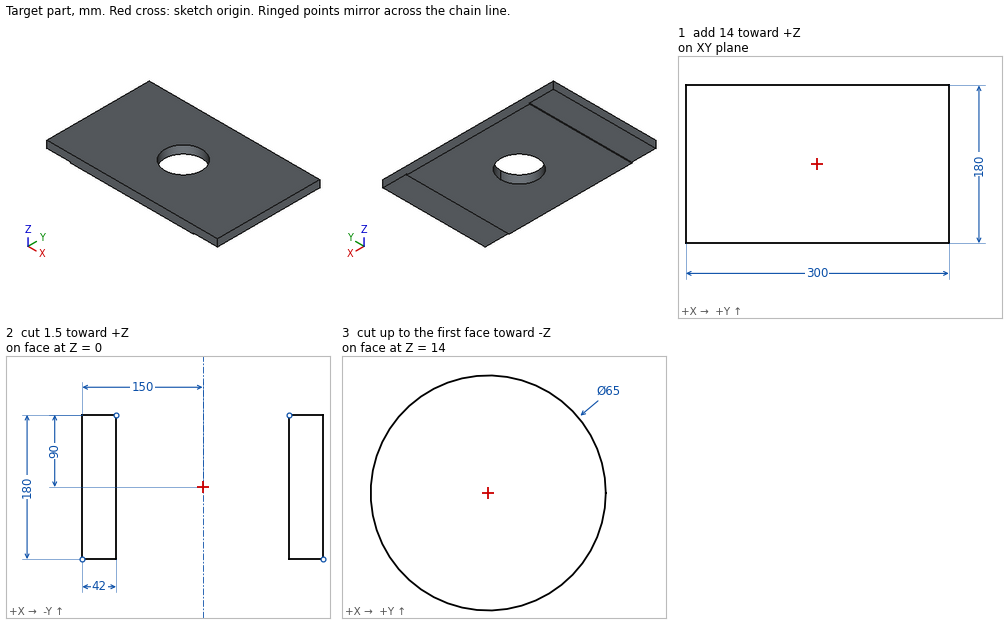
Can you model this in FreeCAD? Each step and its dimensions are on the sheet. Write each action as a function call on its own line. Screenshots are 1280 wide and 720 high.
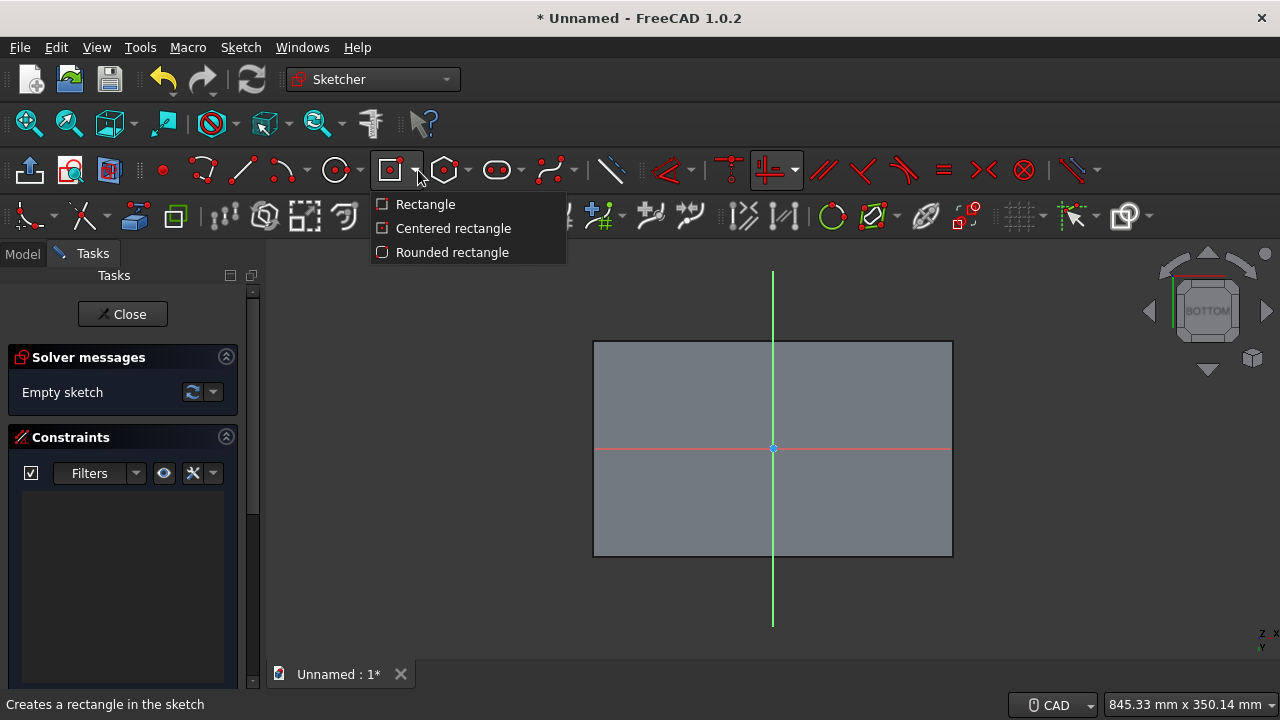
click(468, 204)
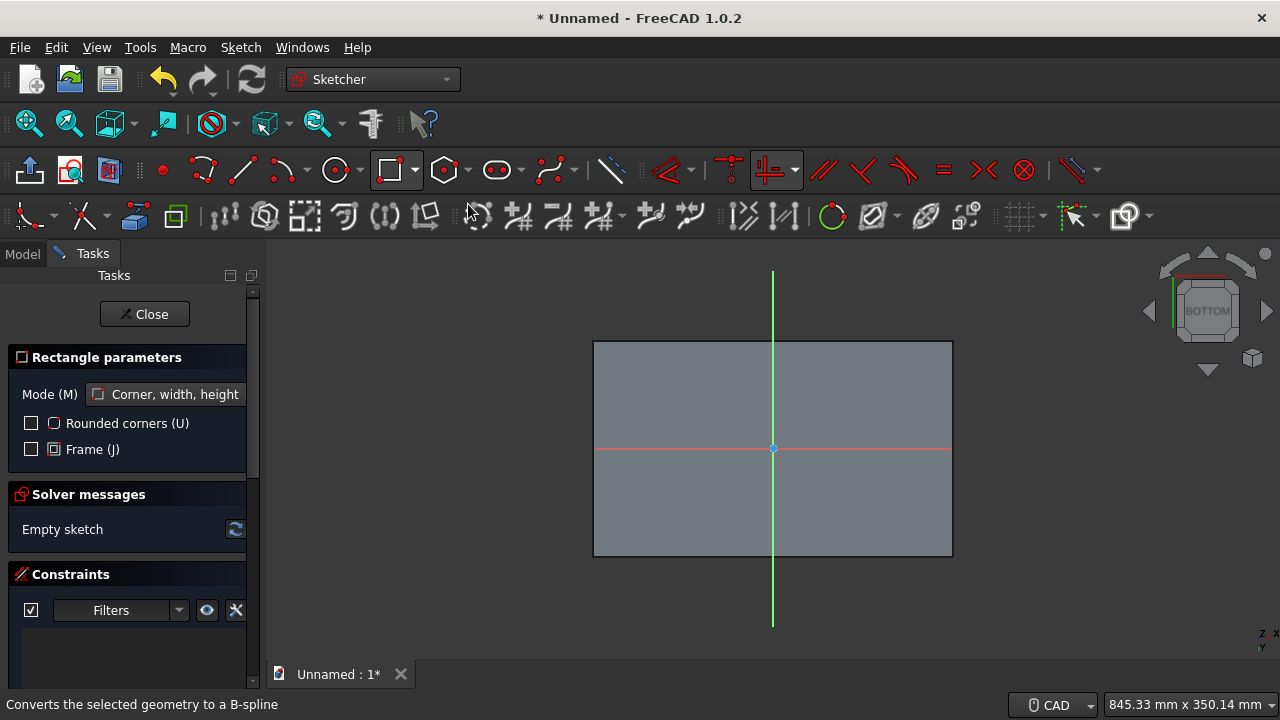
click(593, 341)
click(643, 557)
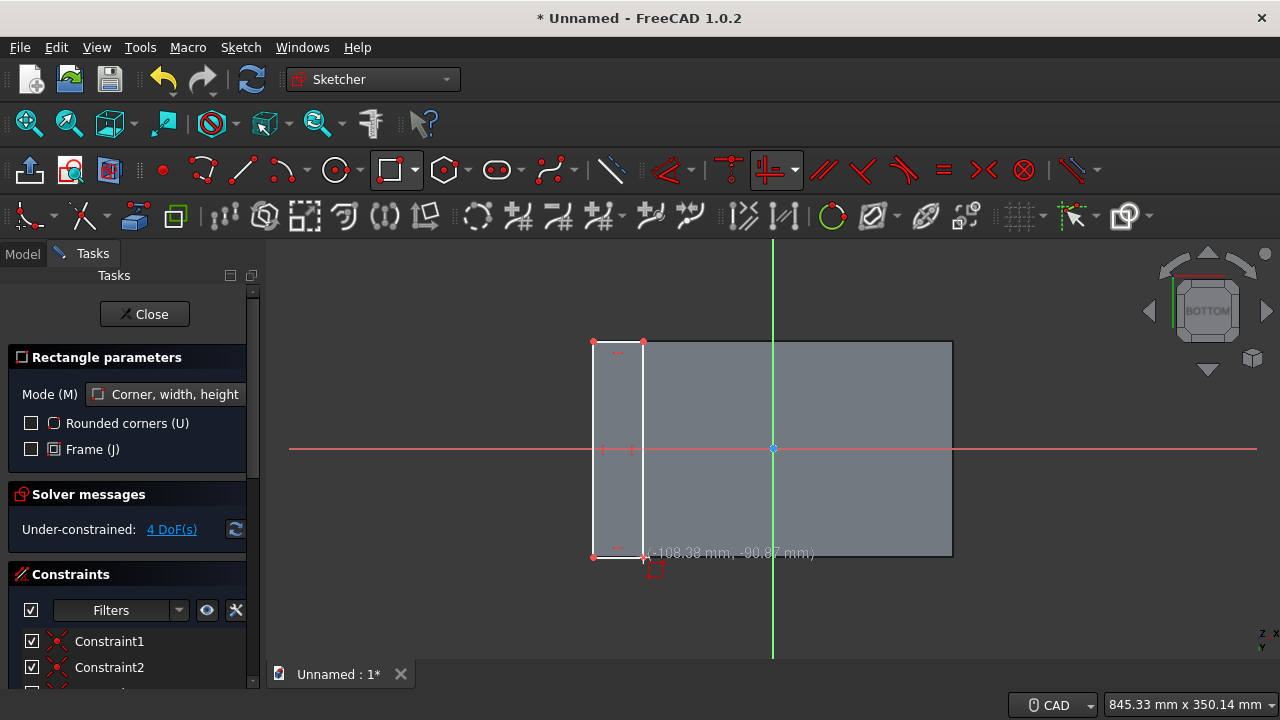
click(903, 341)
click(953, 557)
key(Escape)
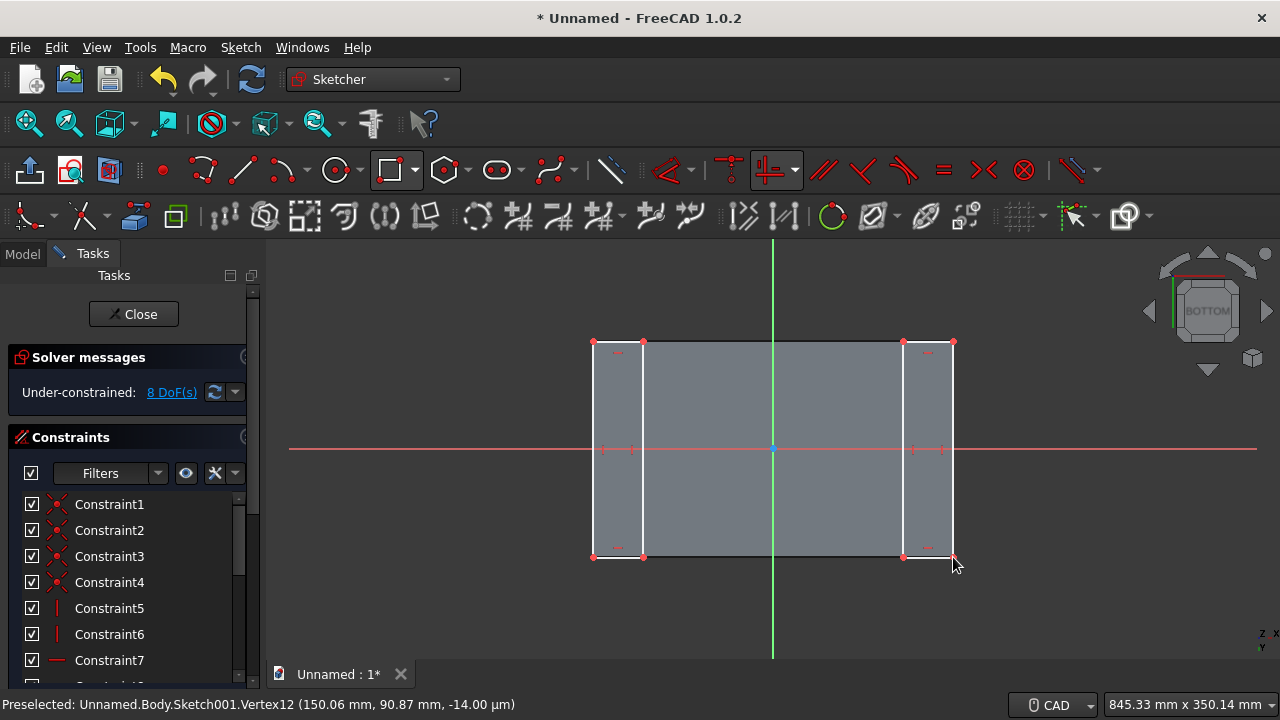
click(643, 342)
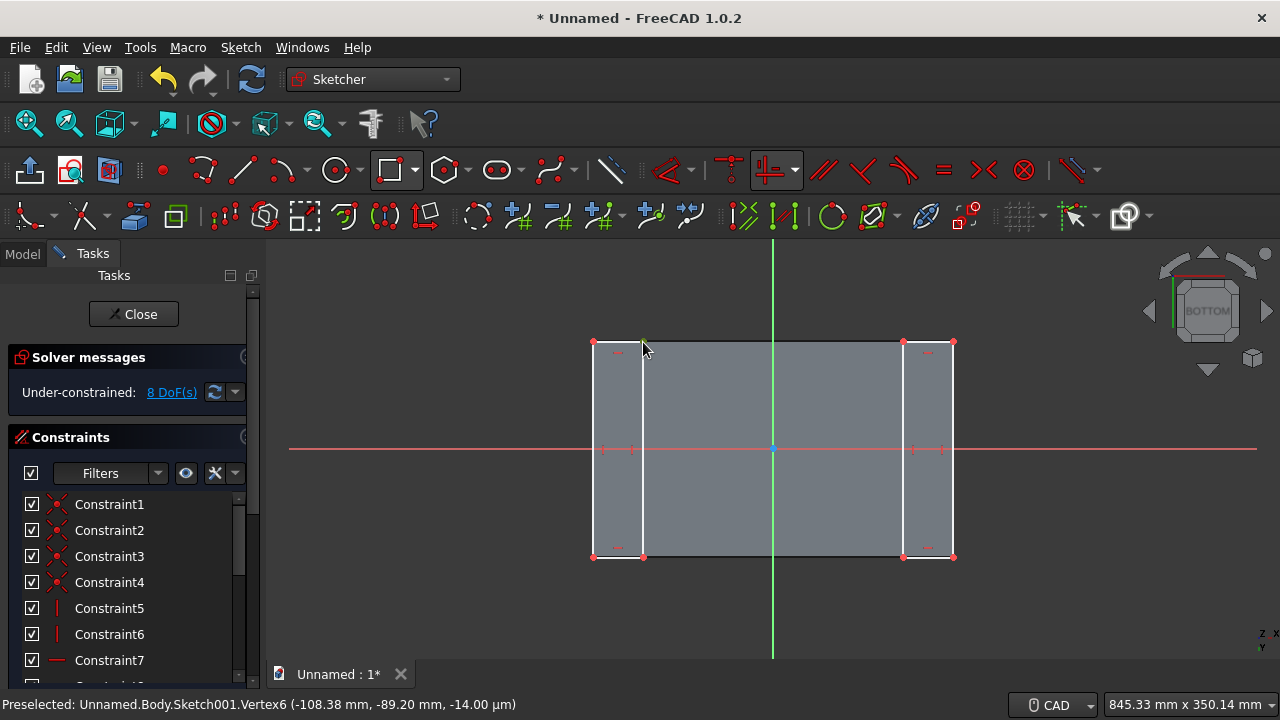
click(903, 342)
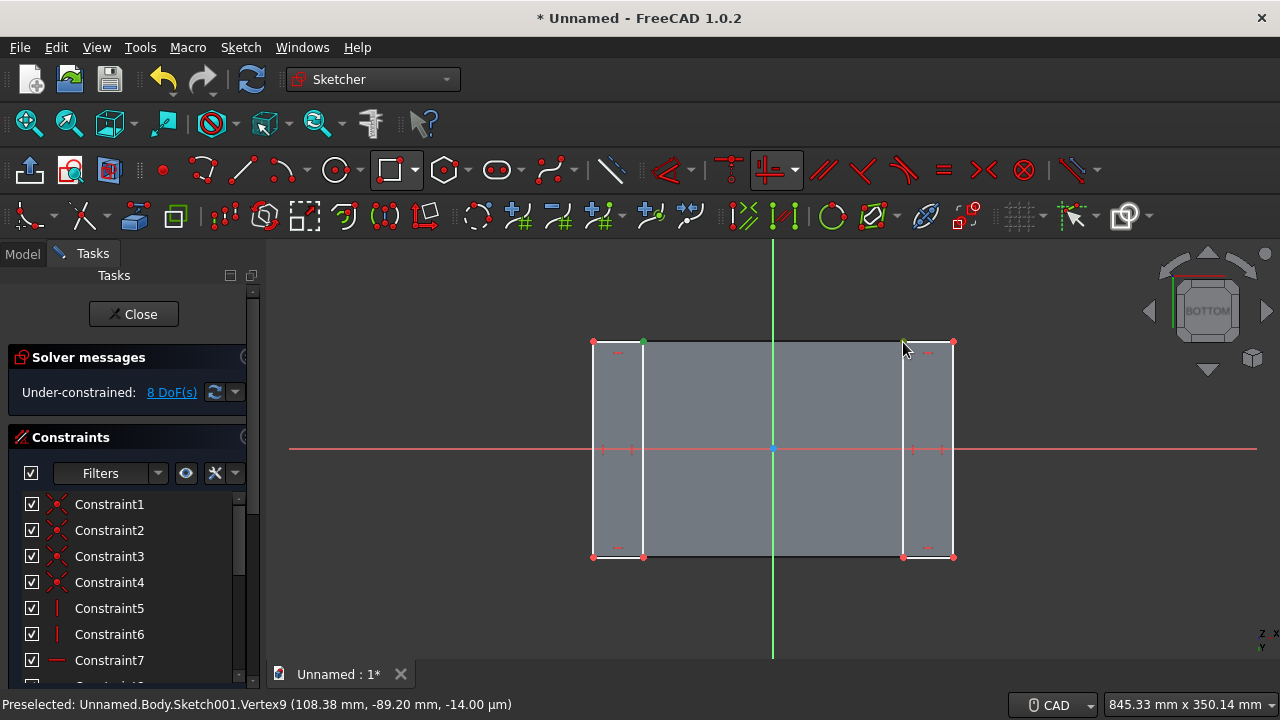
click(773, 605)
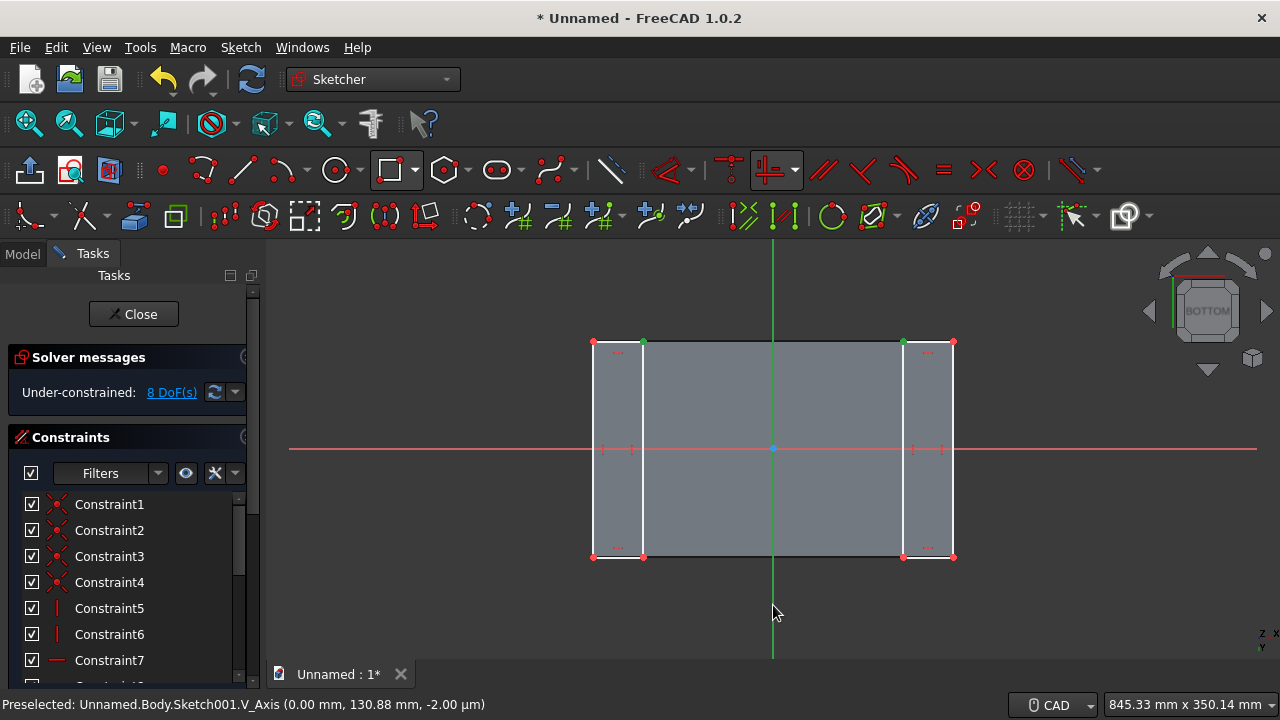
click(984, 170)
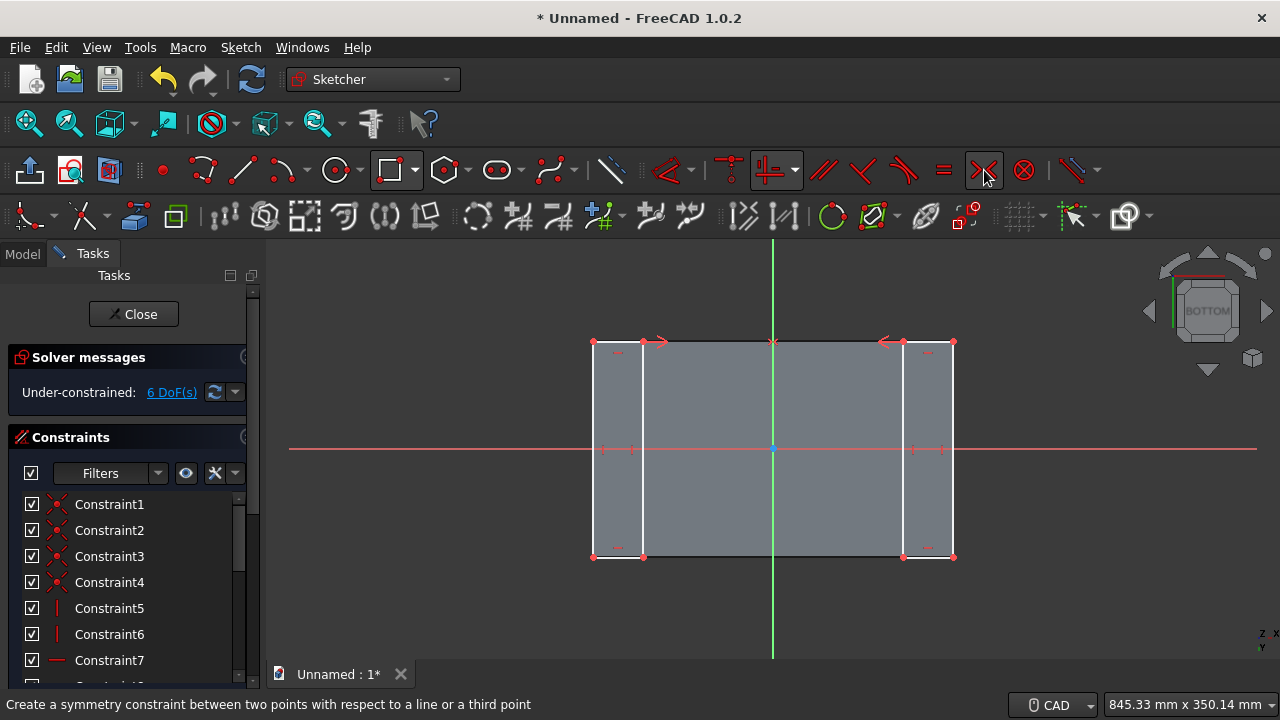
click(593, 558)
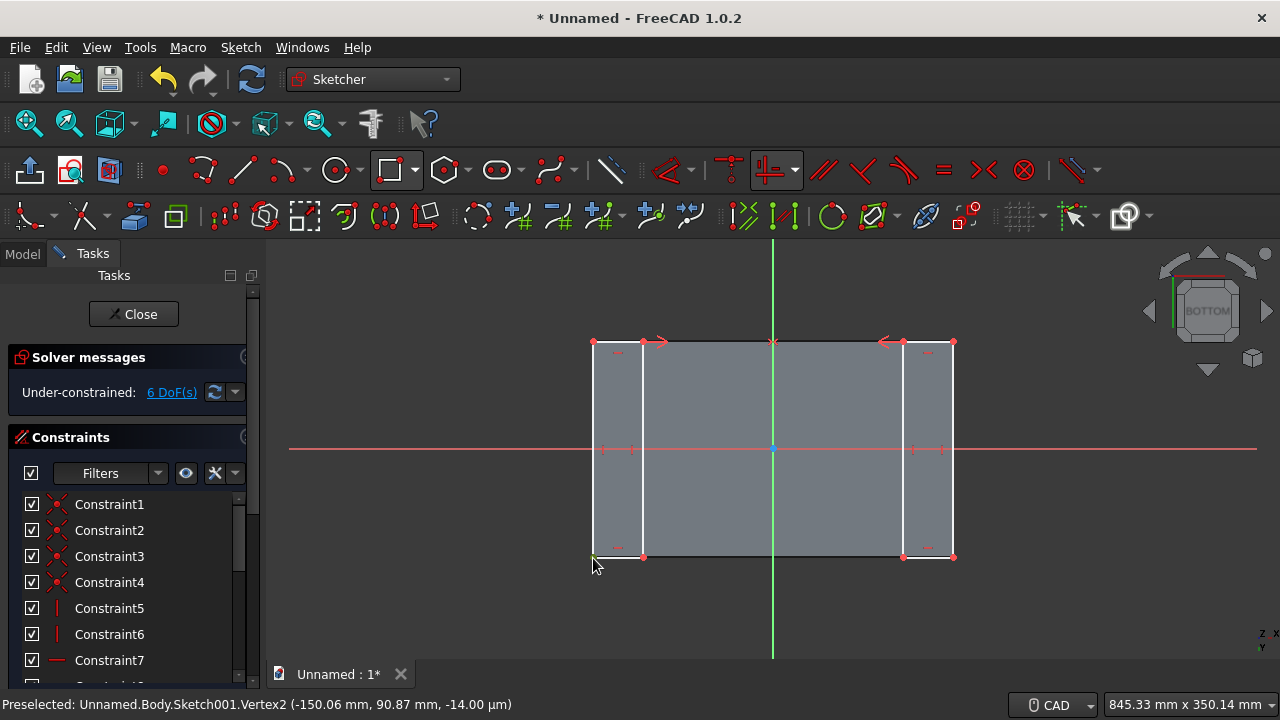
click(953, 558)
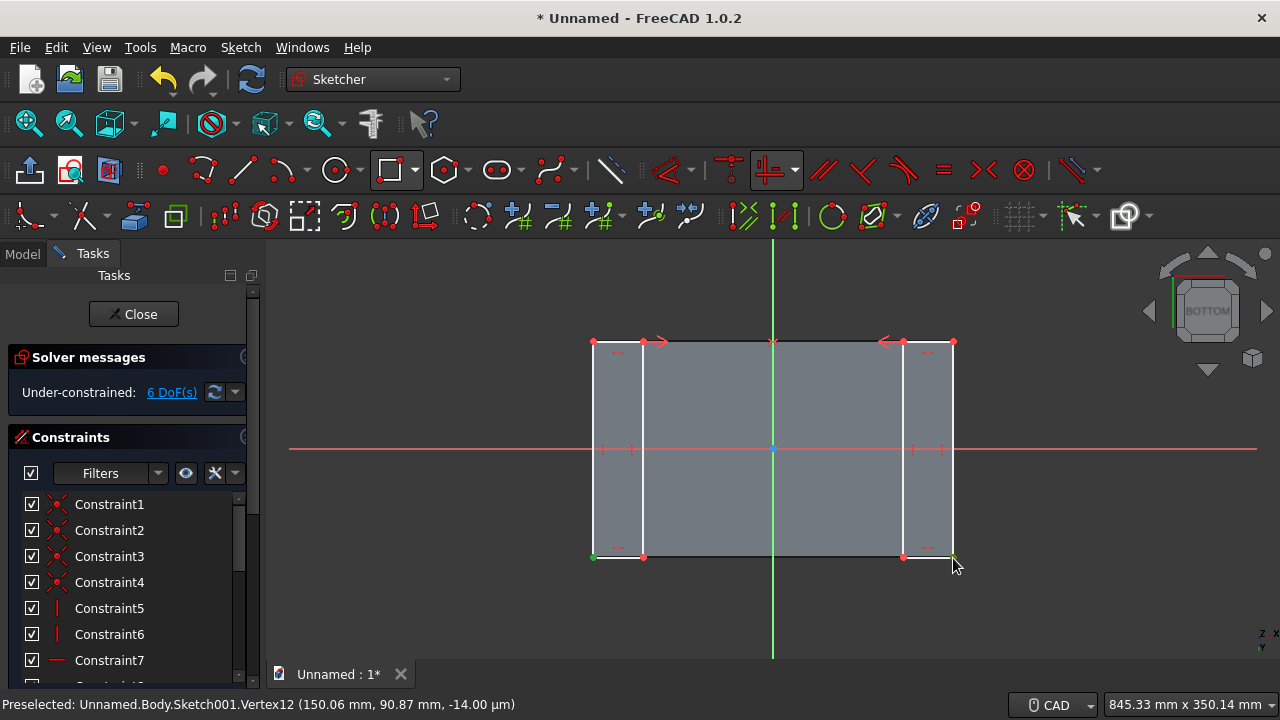
click(773, 605)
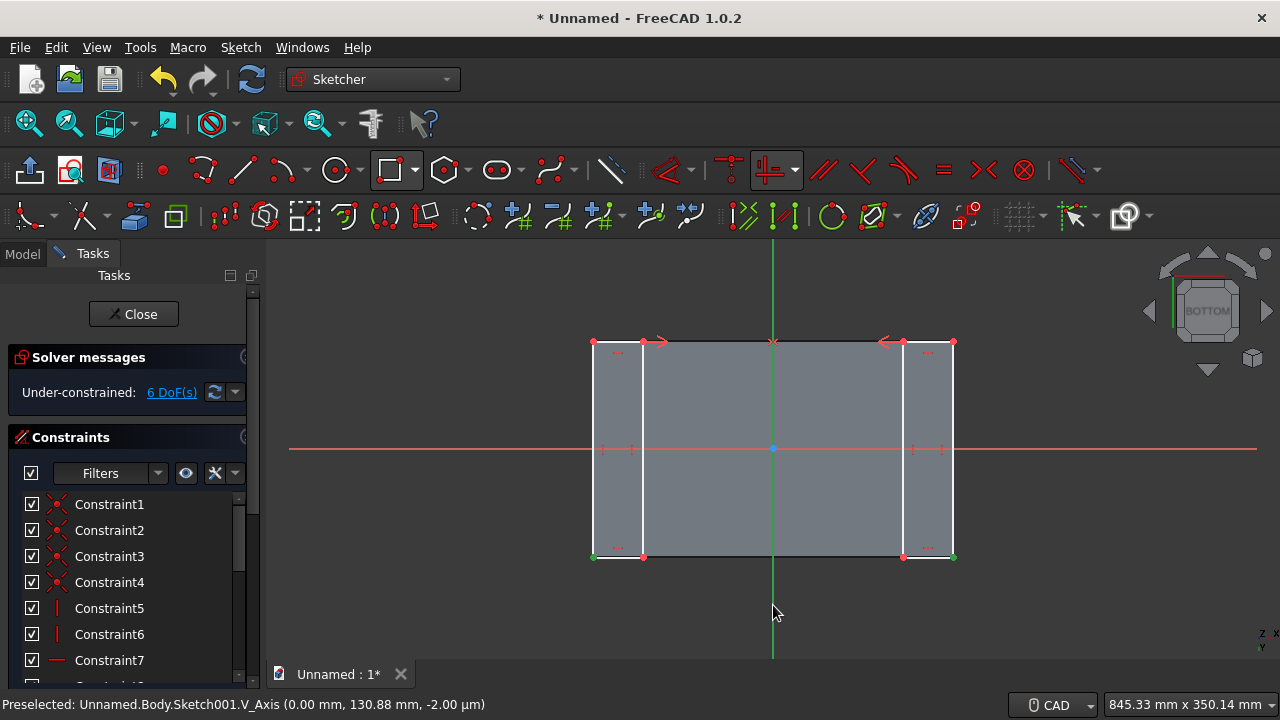
click(984, 170)